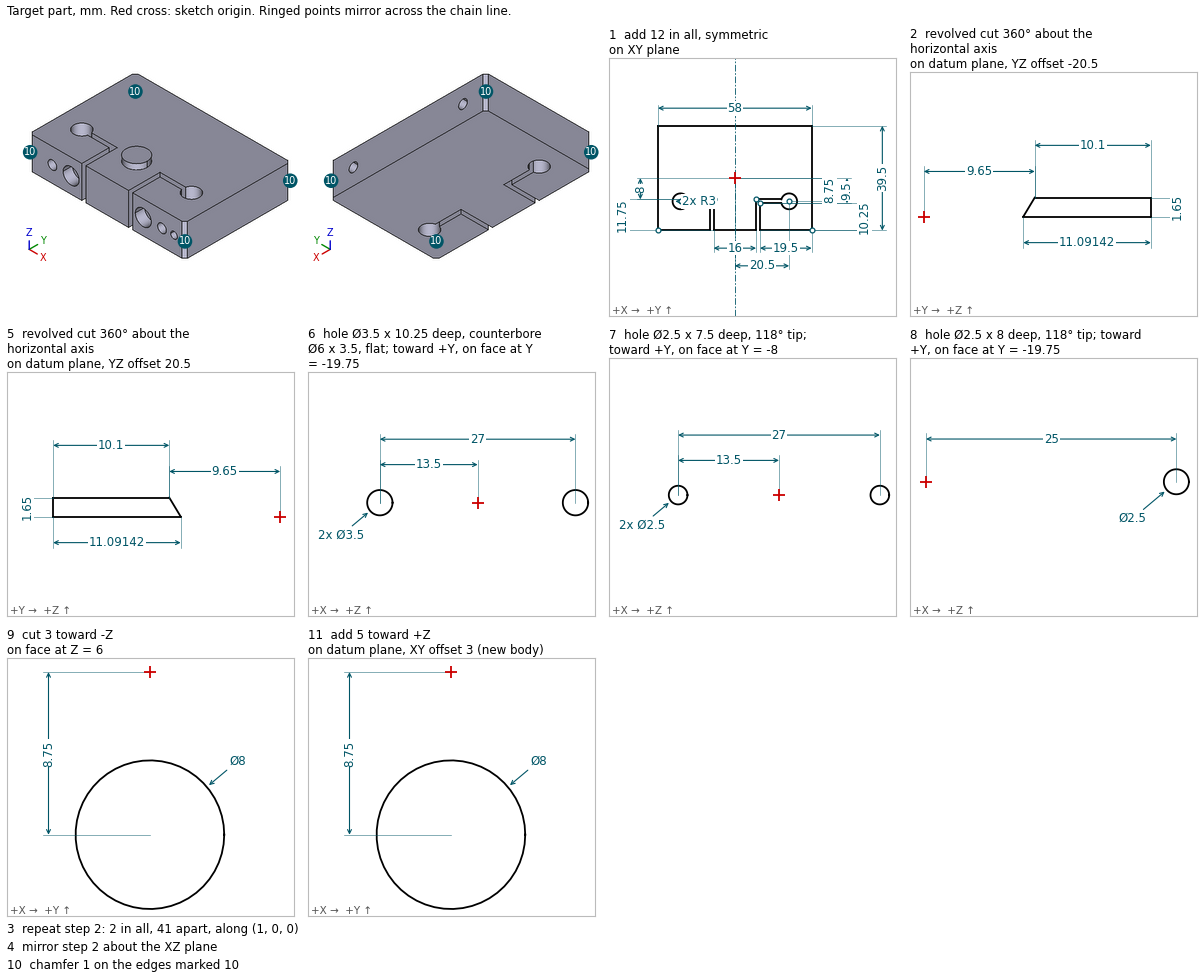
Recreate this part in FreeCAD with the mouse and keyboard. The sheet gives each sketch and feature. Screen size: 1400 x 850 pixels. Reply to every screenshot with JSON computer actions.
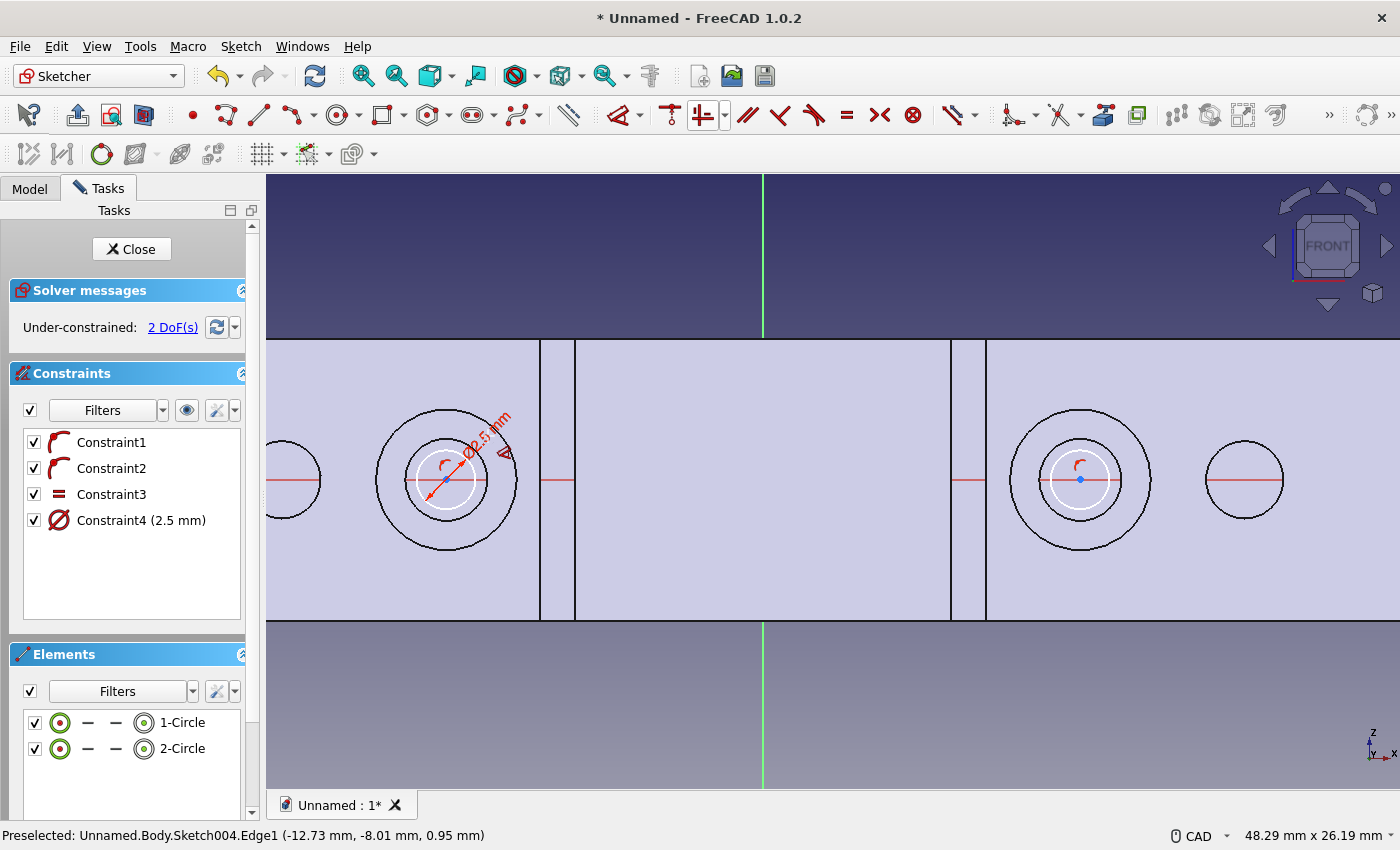
{"action": "left_click", "coordinate": [446, 480]}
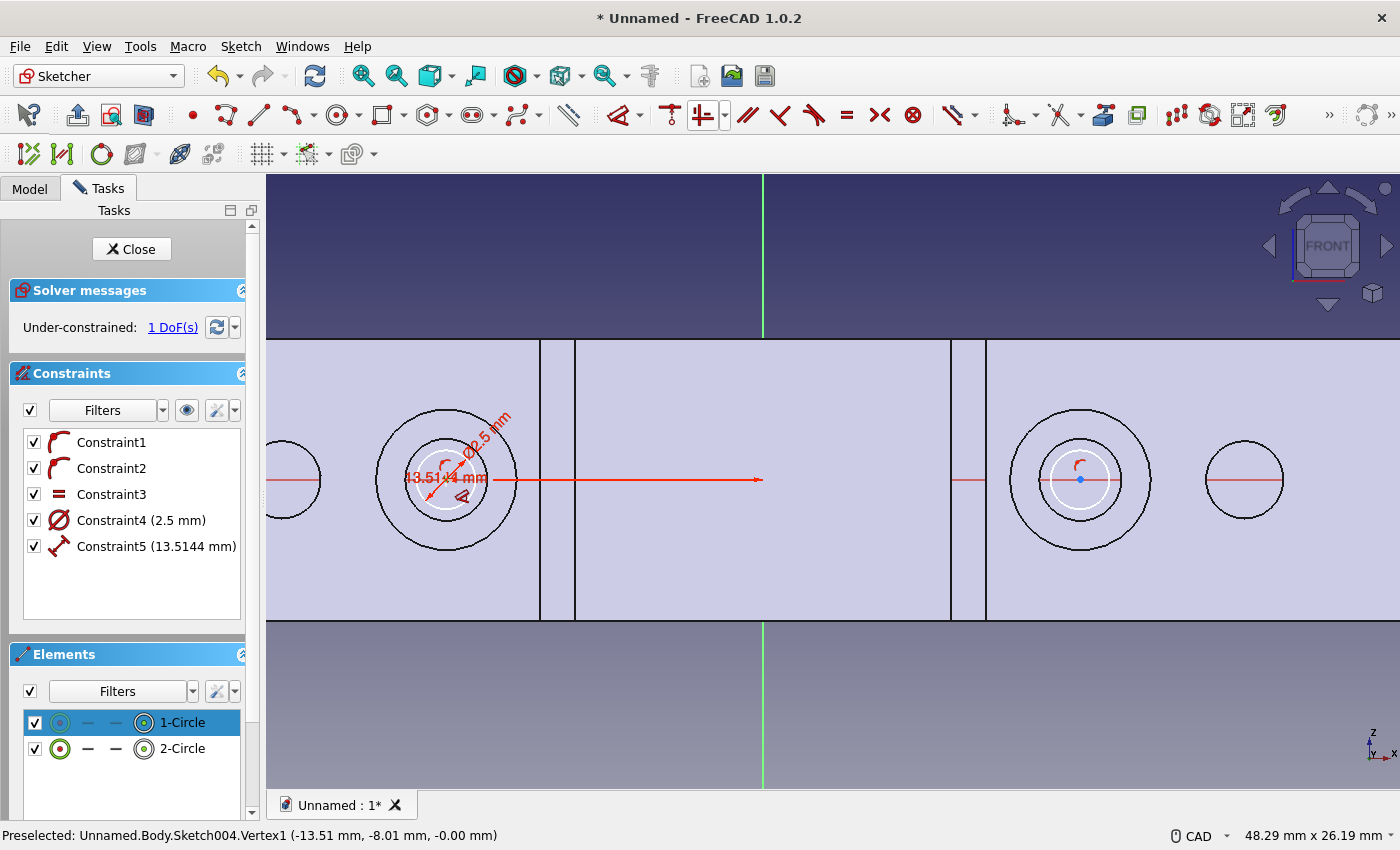
{"action": "left_click", "coordinate": [1080, 480]}
{"action": "left_click", "coordinate": [617, 514]}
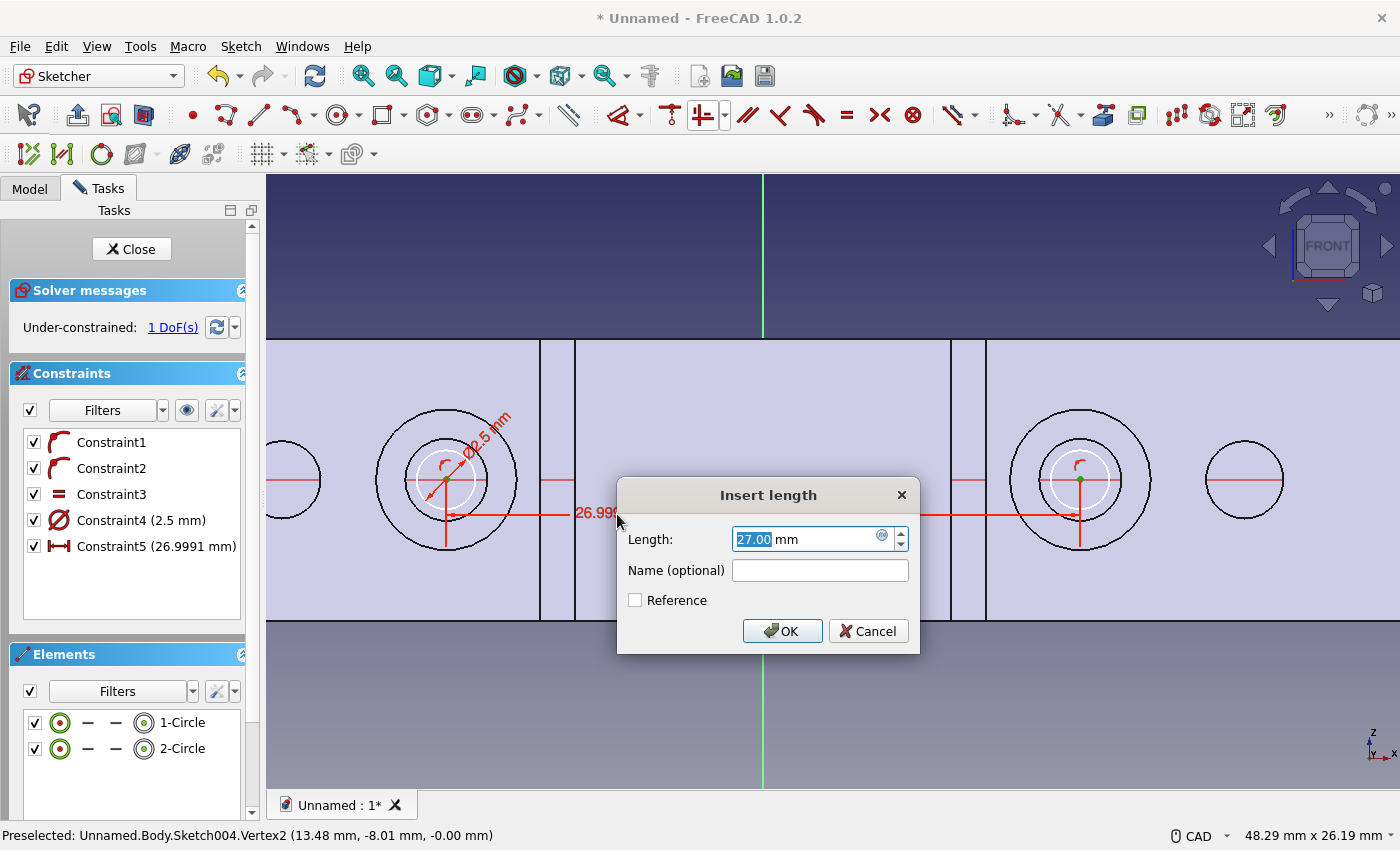
{"action": "type", "text": "27"}
{"action": "key", "text": "Return"}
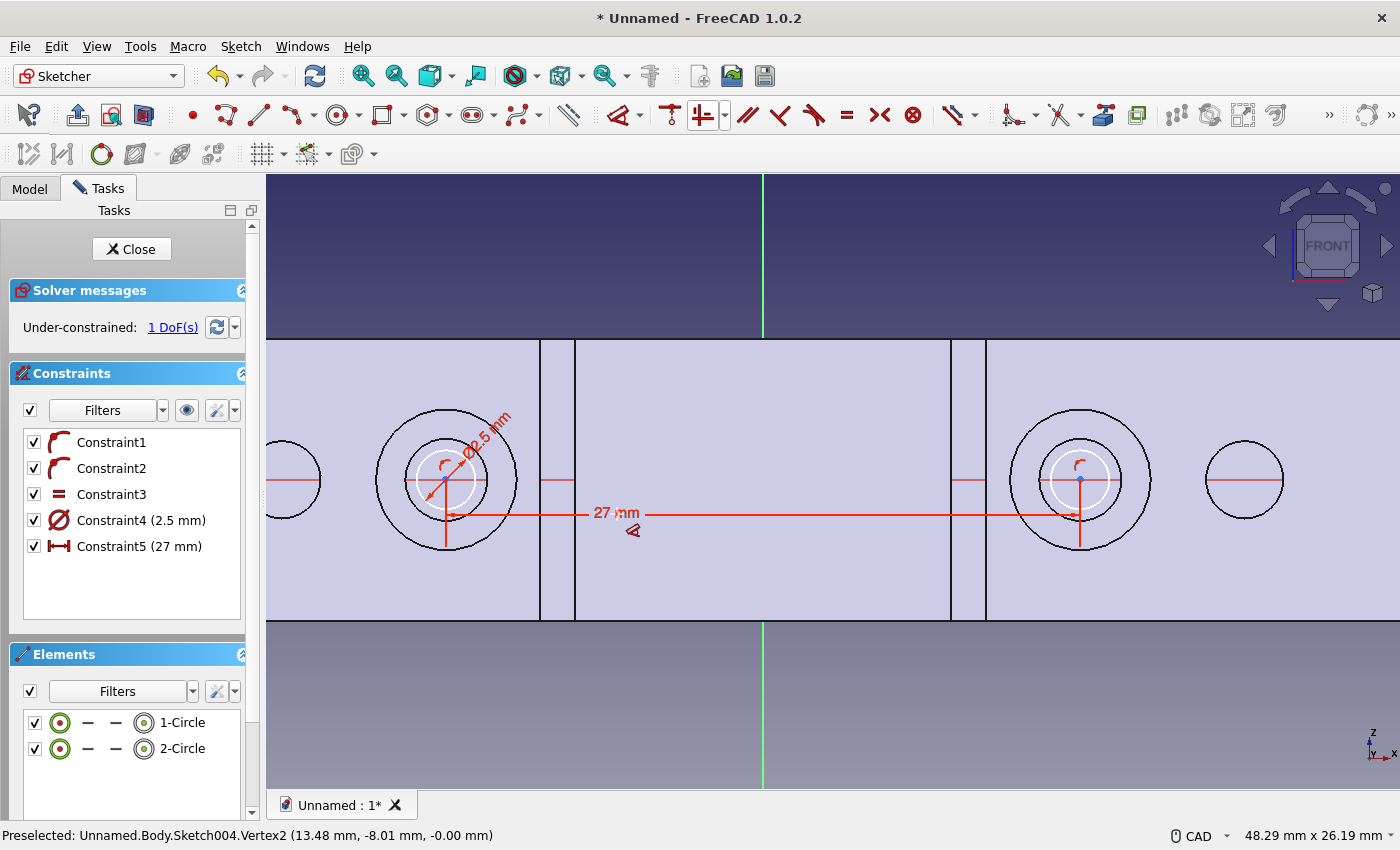
{"action": "left_click", "coordinate": [446, 480]}
{"action": "left_click", "coordinate": [532, 514]}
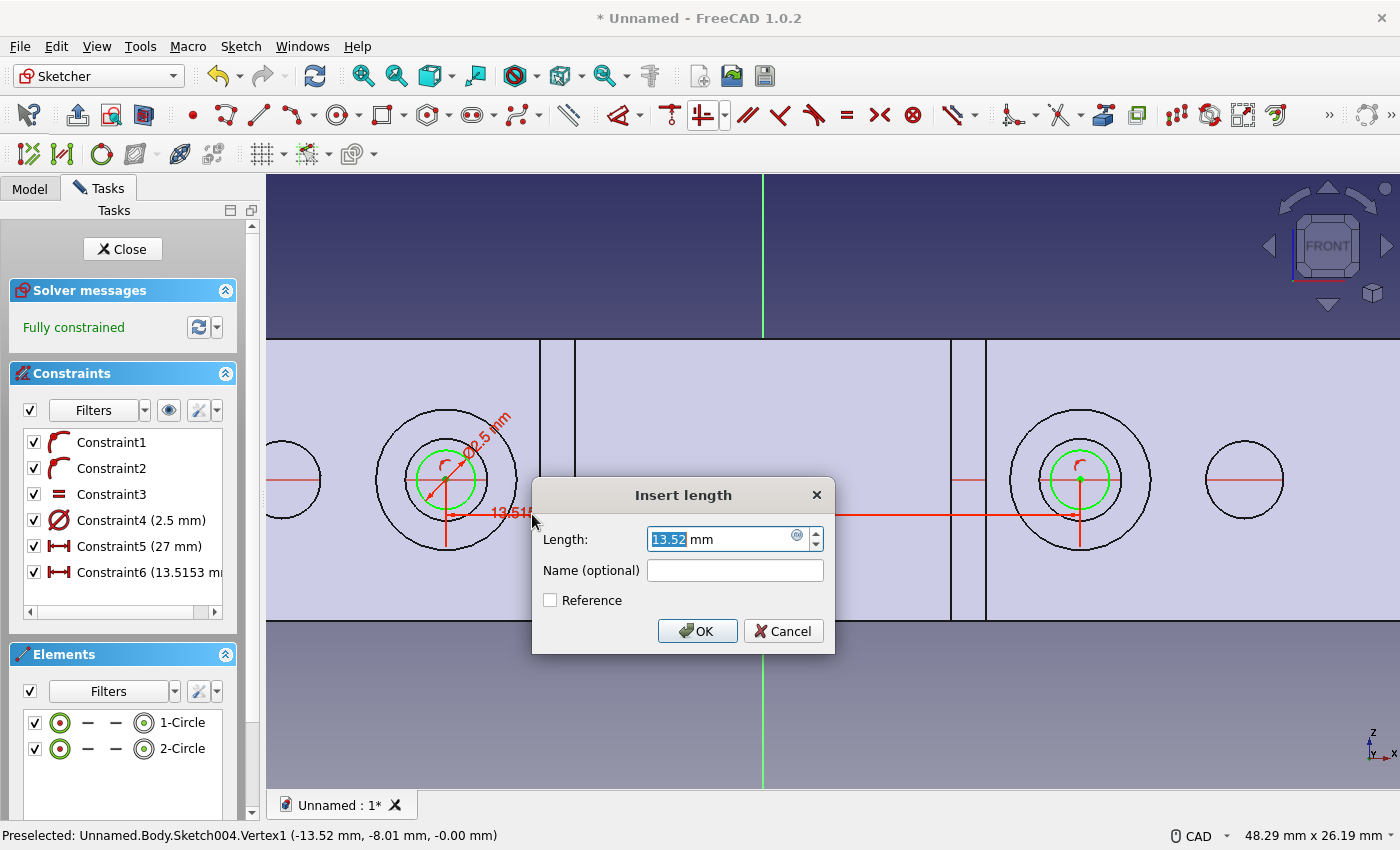
{"action": "type", "text": "13.5"}
{"action": "key", "text": "Return"}
{"action": "key", "text": "Escape"}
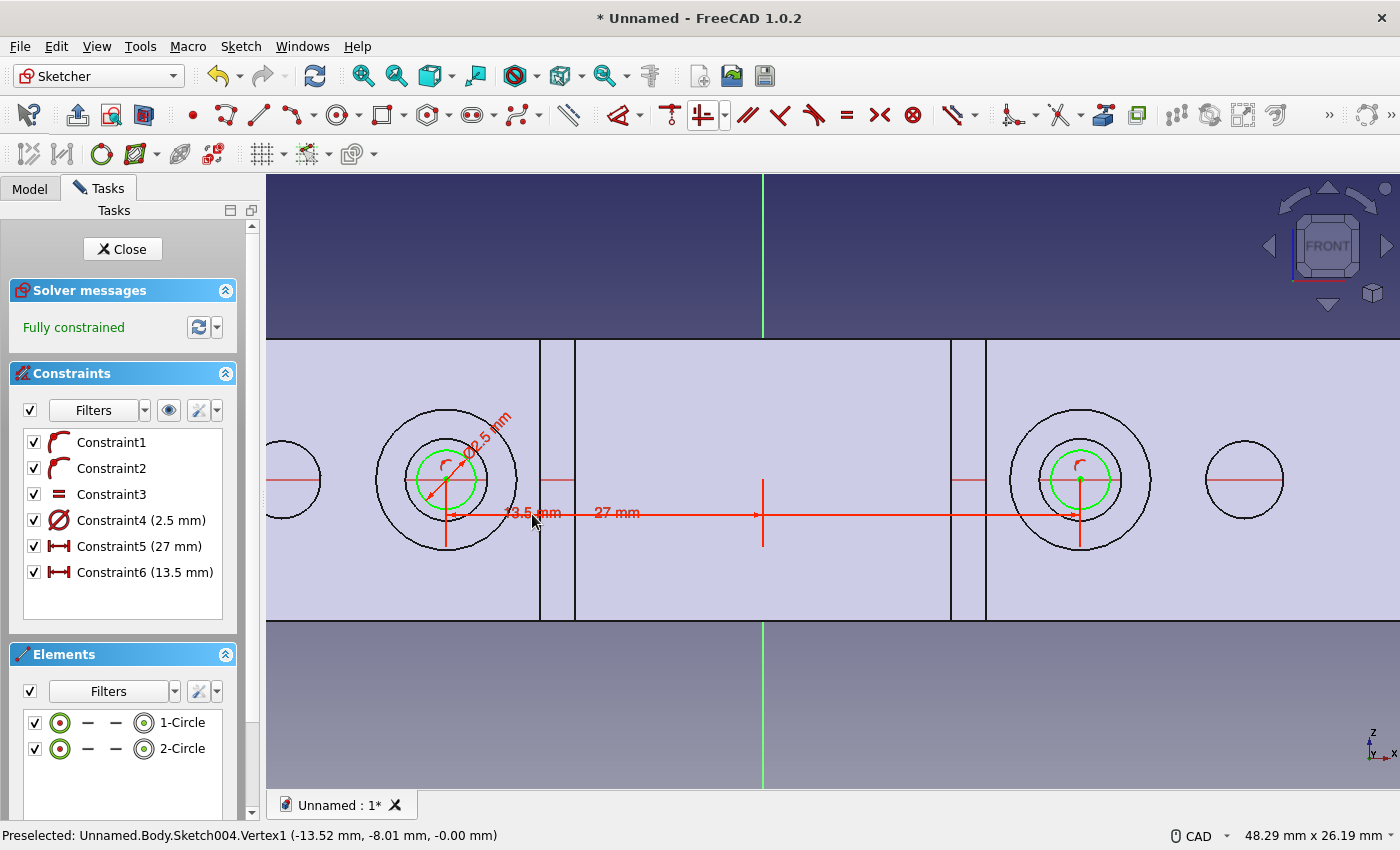
{"action": "left_click", "coordinate": [123, 249]}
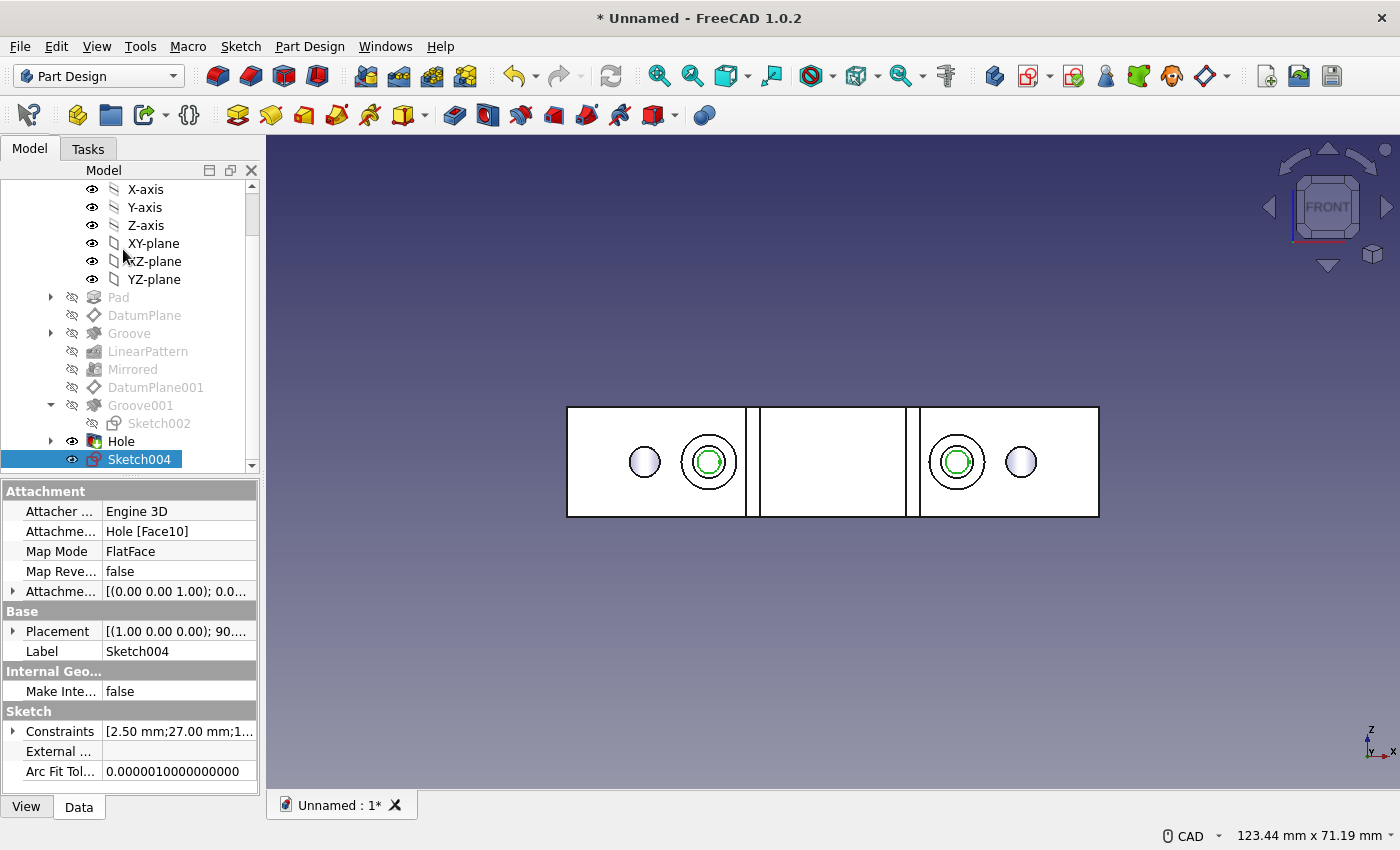
{"action": "left_click", "coordinate": [488, 116]}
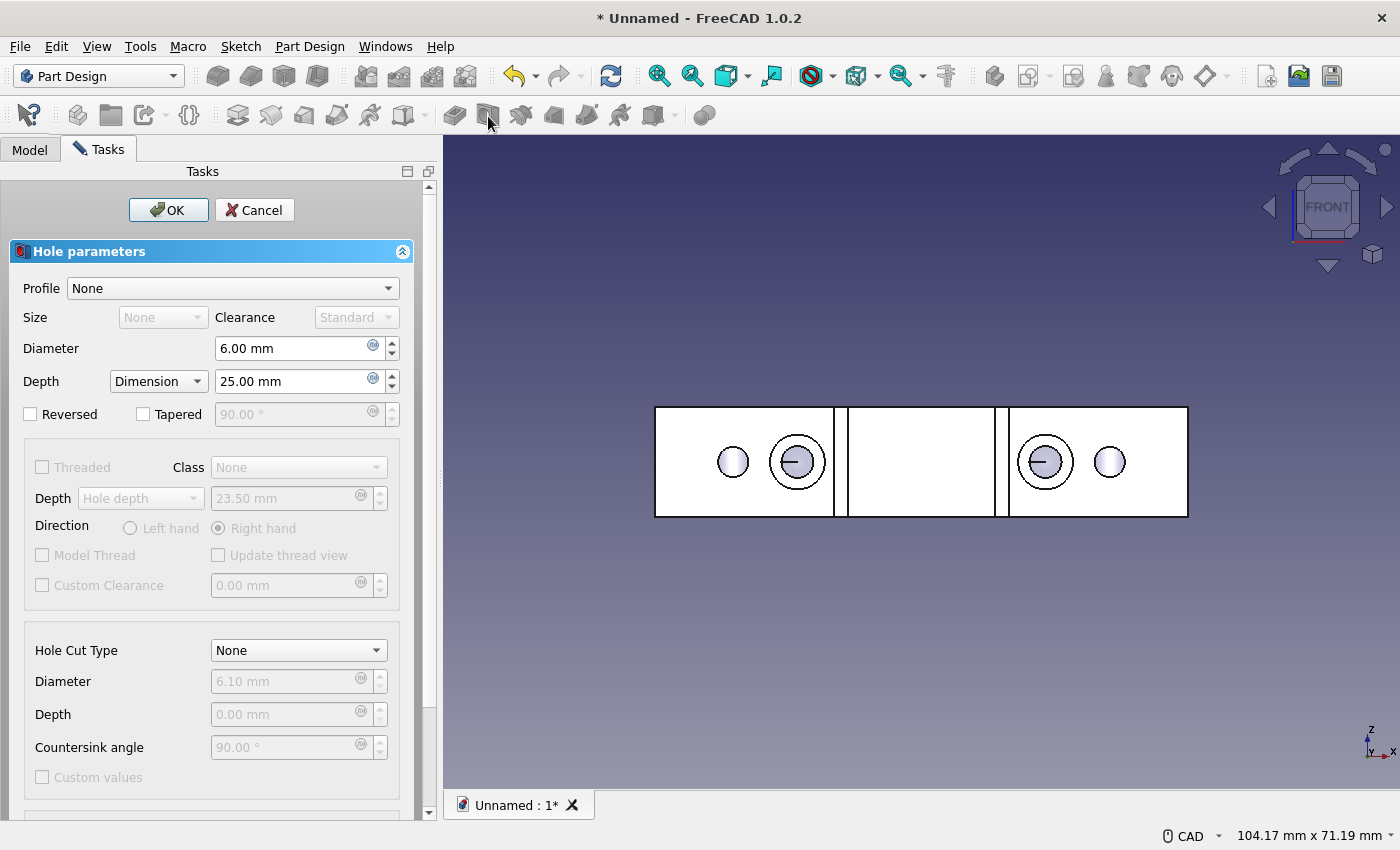
{"action": "triple_click", "coordinate": [300, 348]}